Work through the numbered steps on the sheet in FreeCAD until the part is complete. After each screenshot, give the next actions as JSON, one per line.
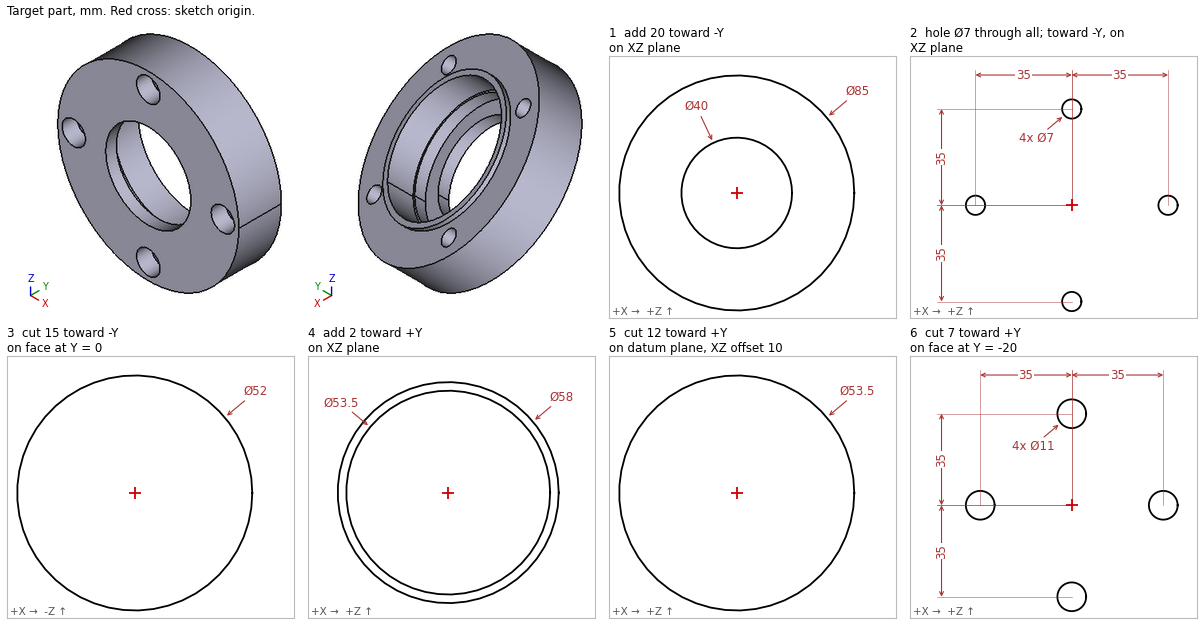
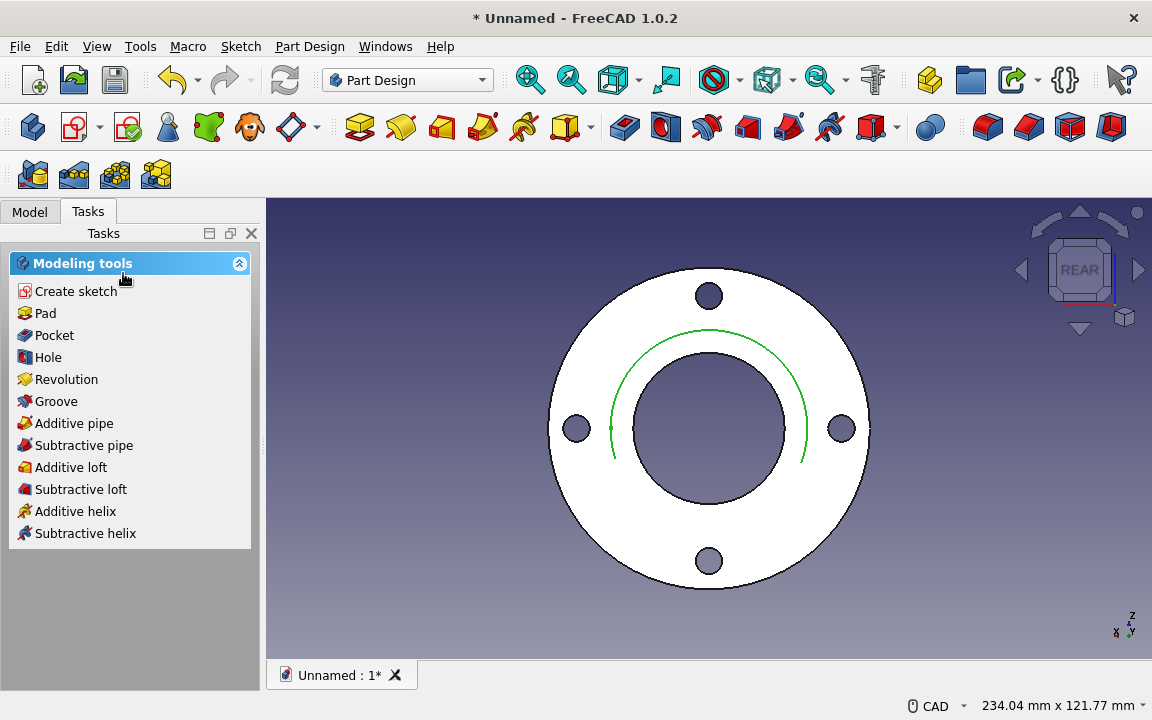
{"action": "left_click", "coordinate": [625, 128]}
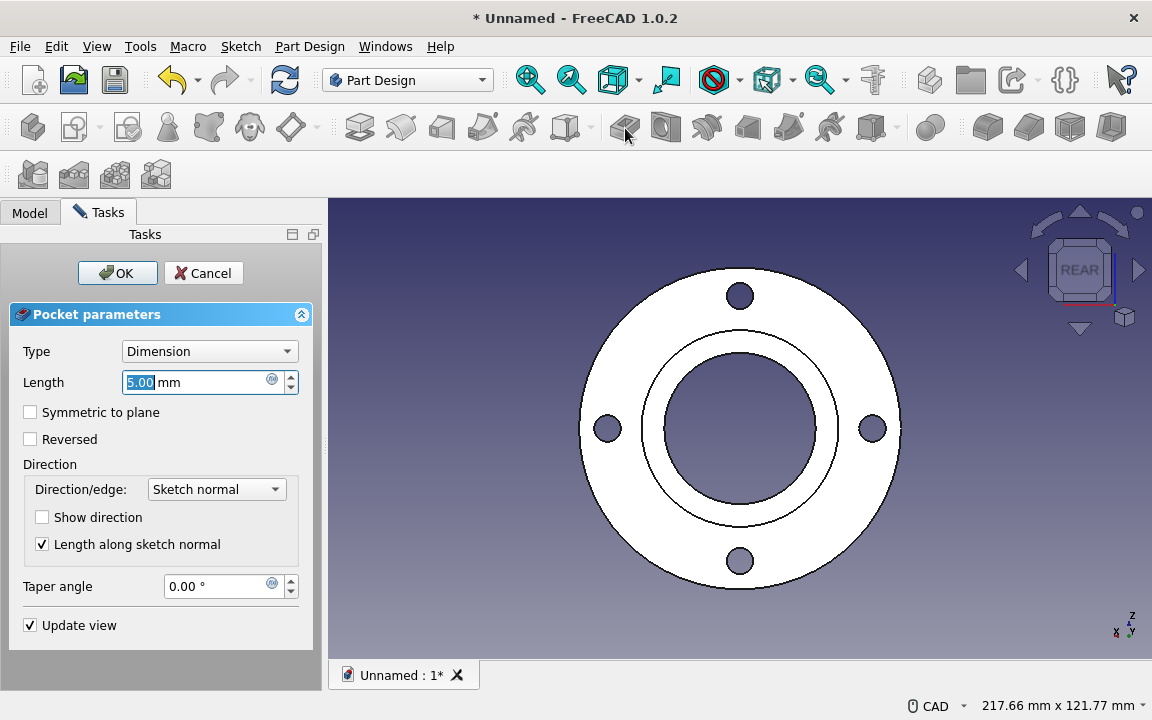
{"action": "type", "text": "15"}
{"action": "key", "text": "Tab"}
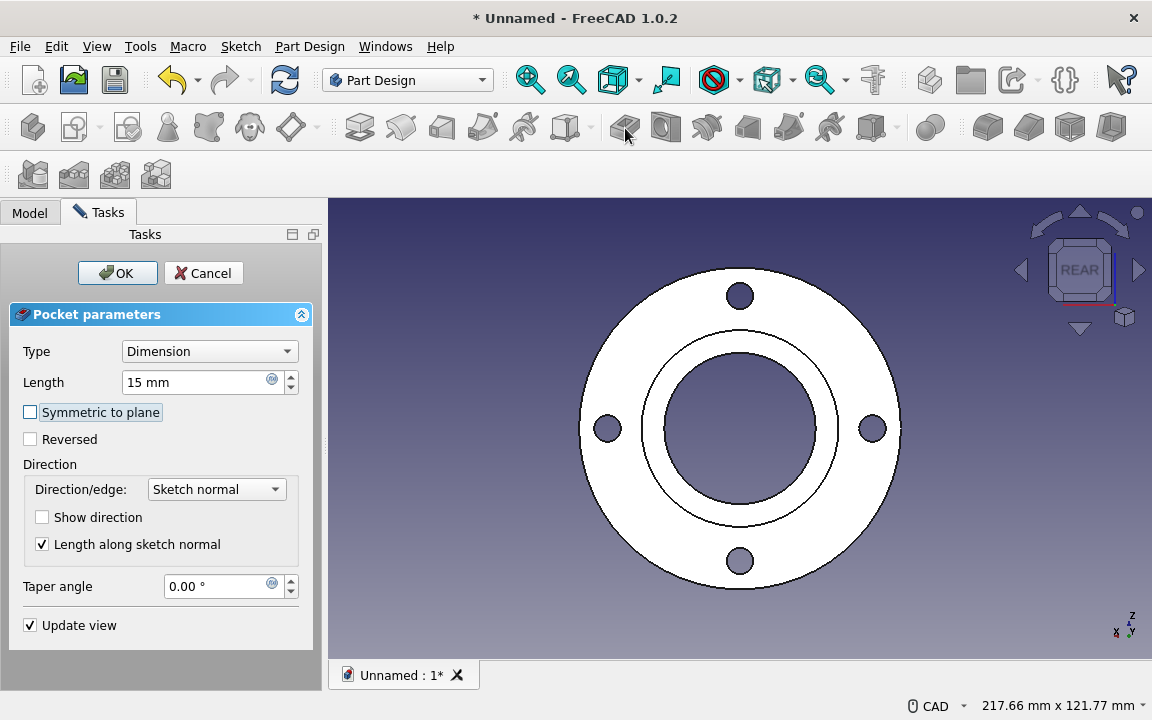
{"action": "left_click", "coordinate": [118, 273]}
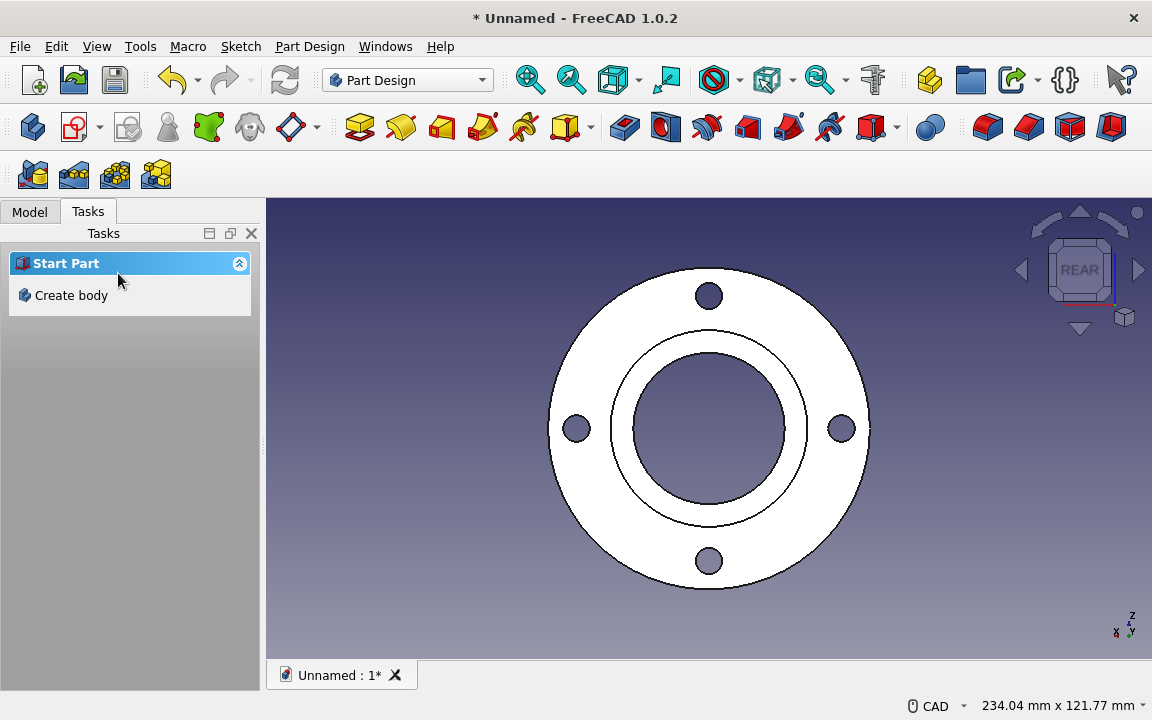
{"action": "left_click", "coordinate": [74, 128]}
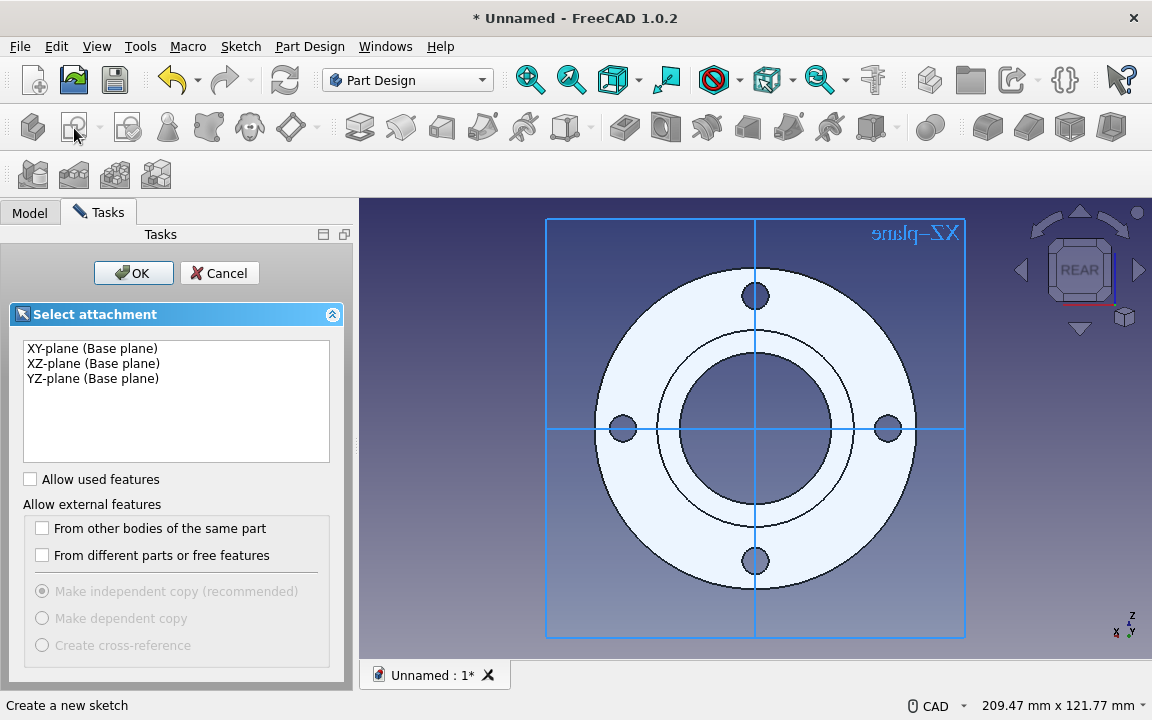
{"action": "left_click", "coordinate": [84, 364]}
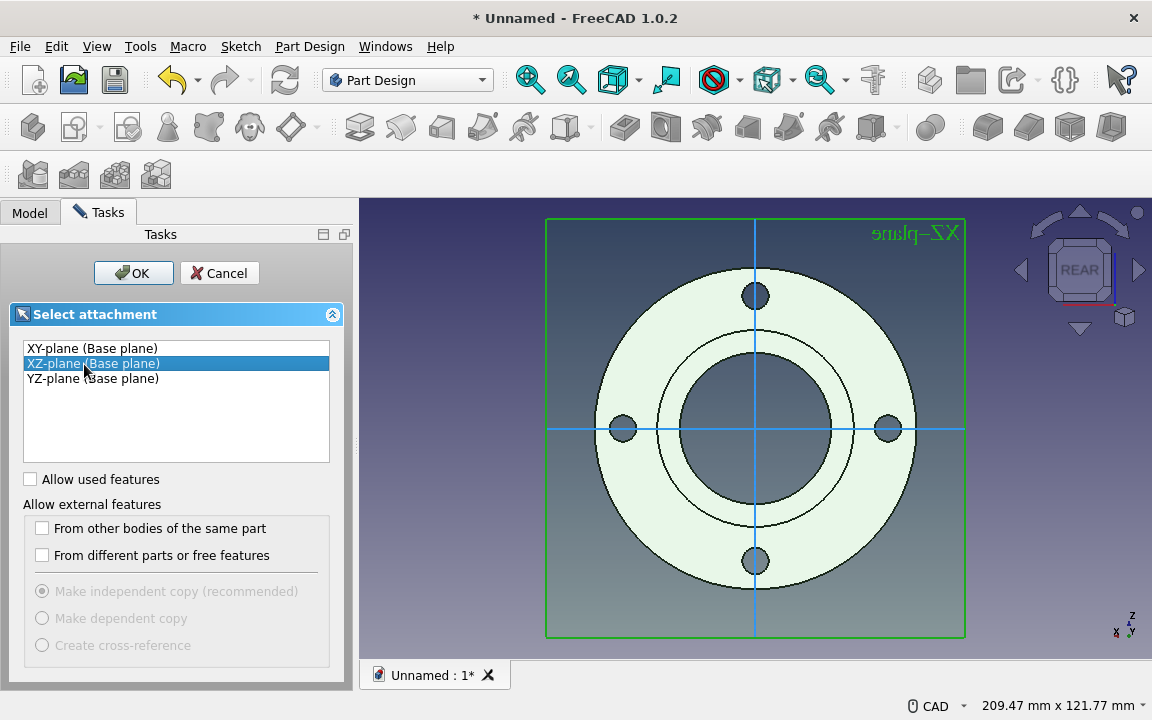
{"action": "left_click", "coordinate": [134, 273]}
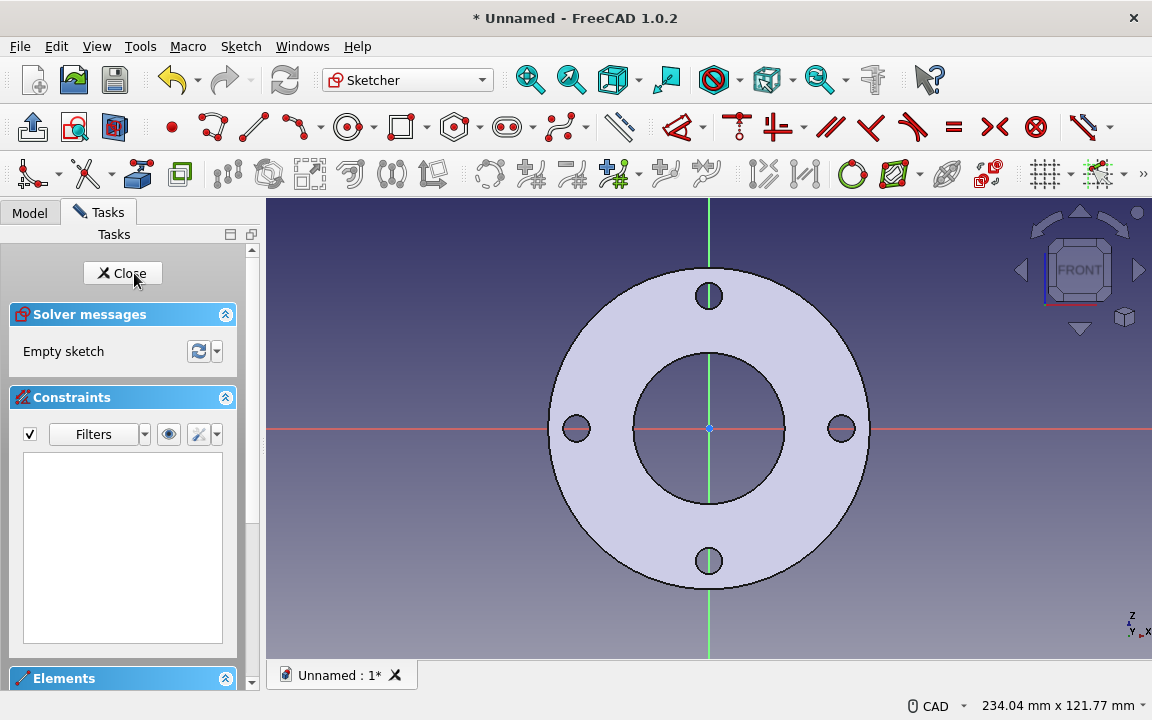
{"action": "left_click", "coordinate": [115, 128]}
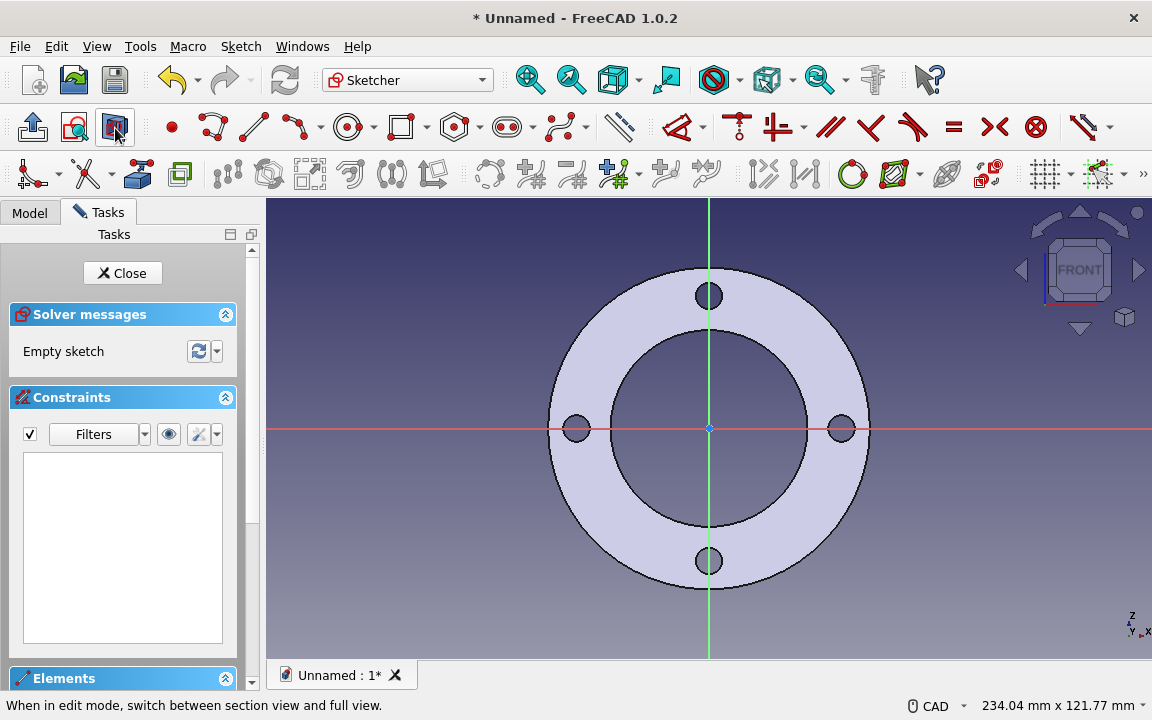
{"action": "left_click", "coordinate": [348, 128]}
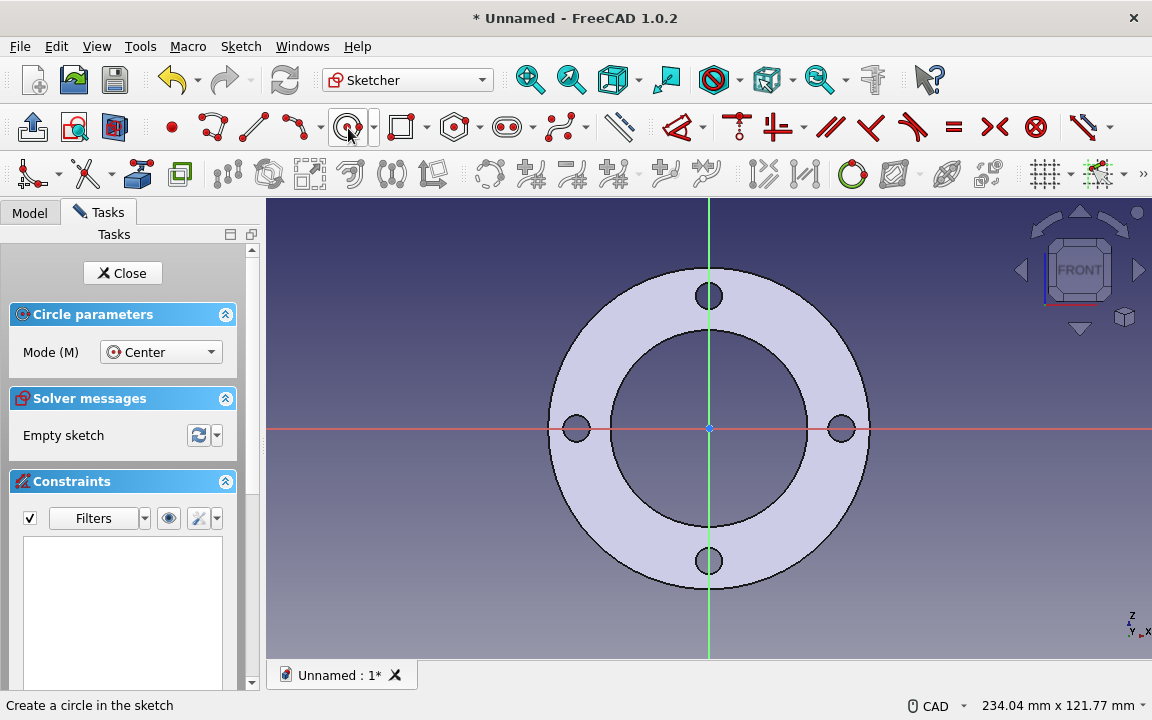
{"action": "left_click", "coordinate": [709, 429]}
{"action": "mouse_move", "coordinate": [787, 351]}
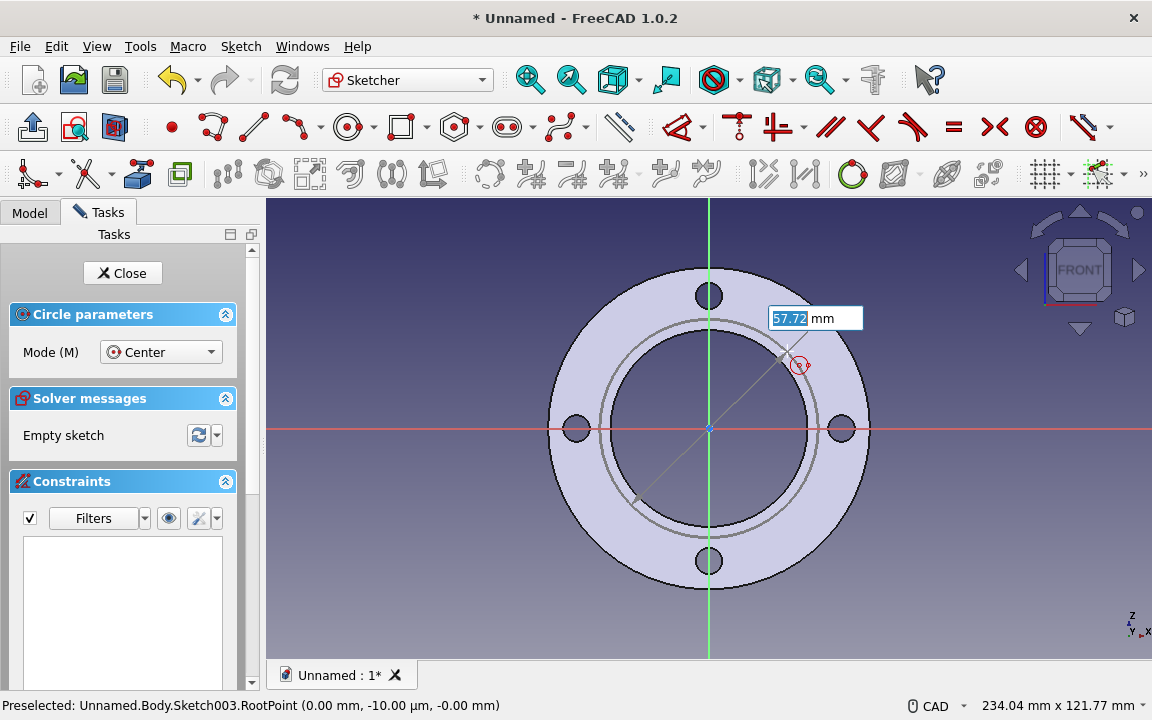
{"action": "type", "text": "58"}
{"action": "key", "text": "Return"}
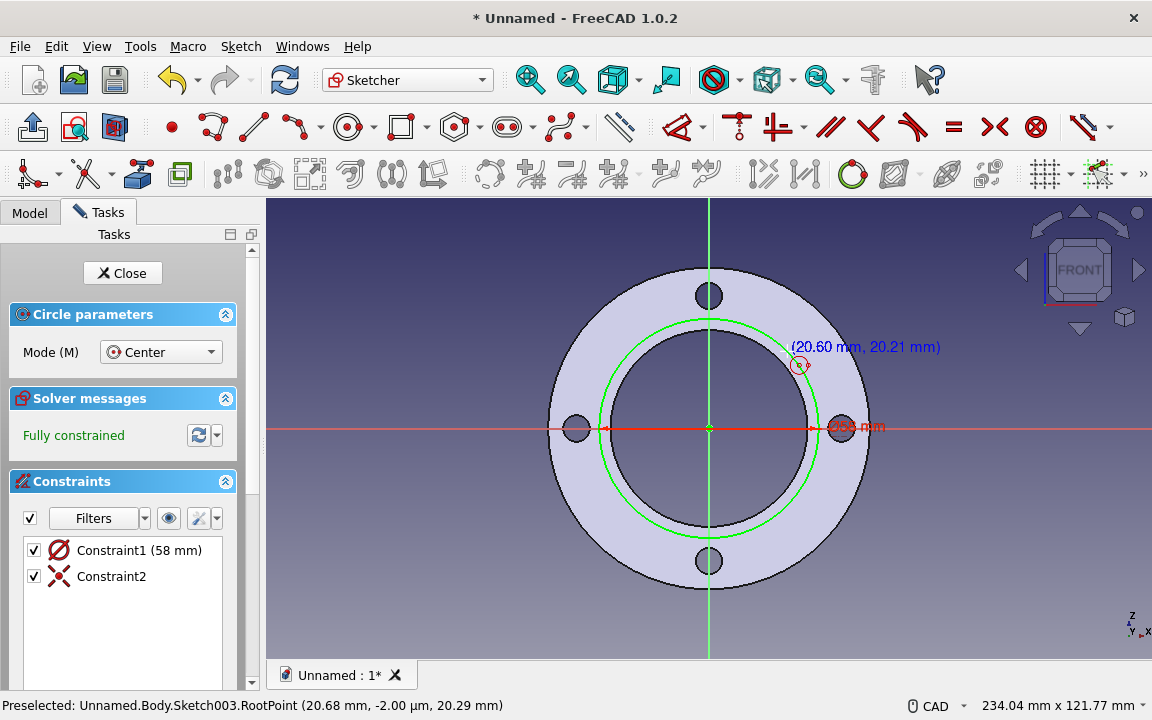
{"action": "left_click", "coordinate": [709, 429]}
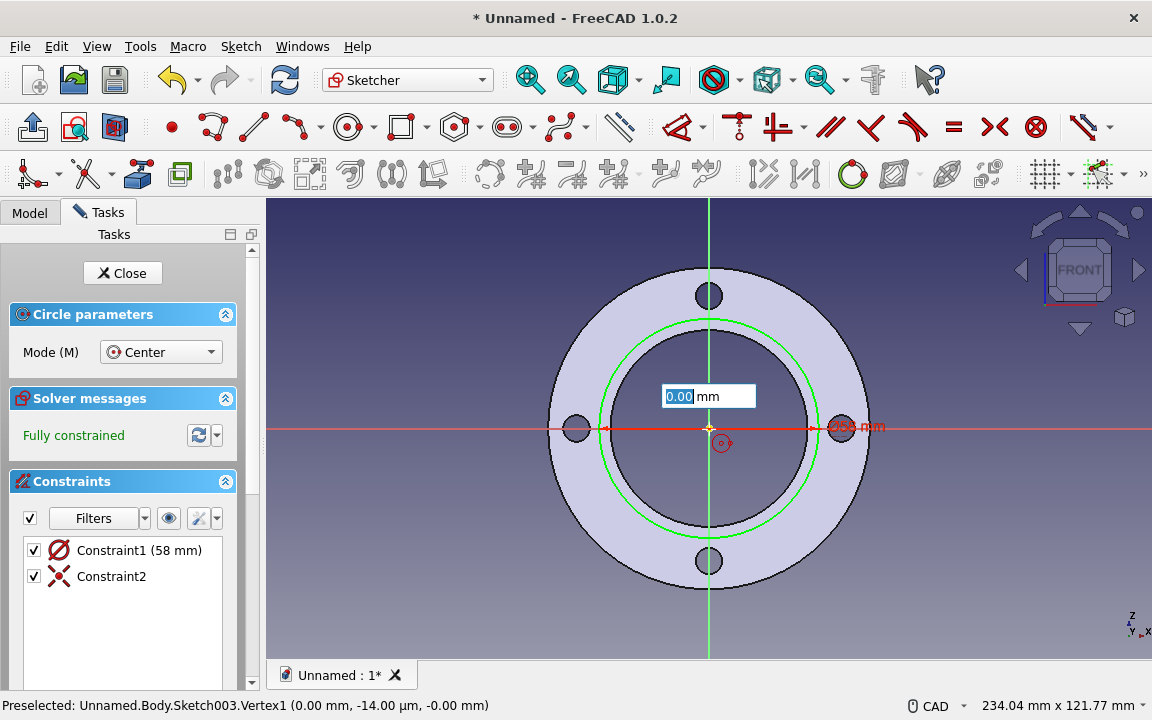
{"action": "scroll", "coordinate": [674, 524], "scroll_direction": "up", "scroll_amount": 4}
{"action": "mouse_move", "coordinate": [674, 522]}